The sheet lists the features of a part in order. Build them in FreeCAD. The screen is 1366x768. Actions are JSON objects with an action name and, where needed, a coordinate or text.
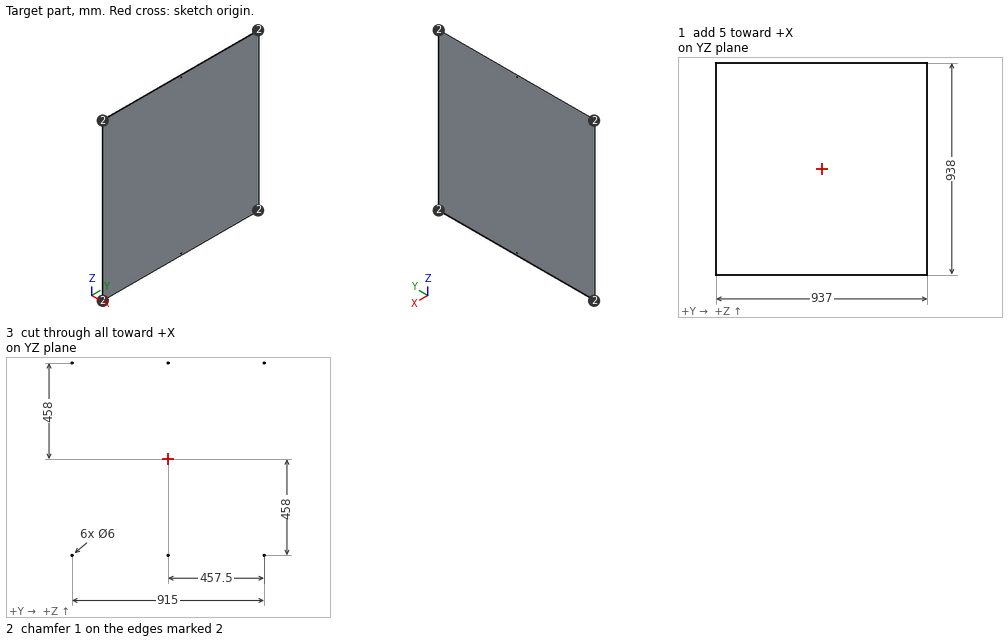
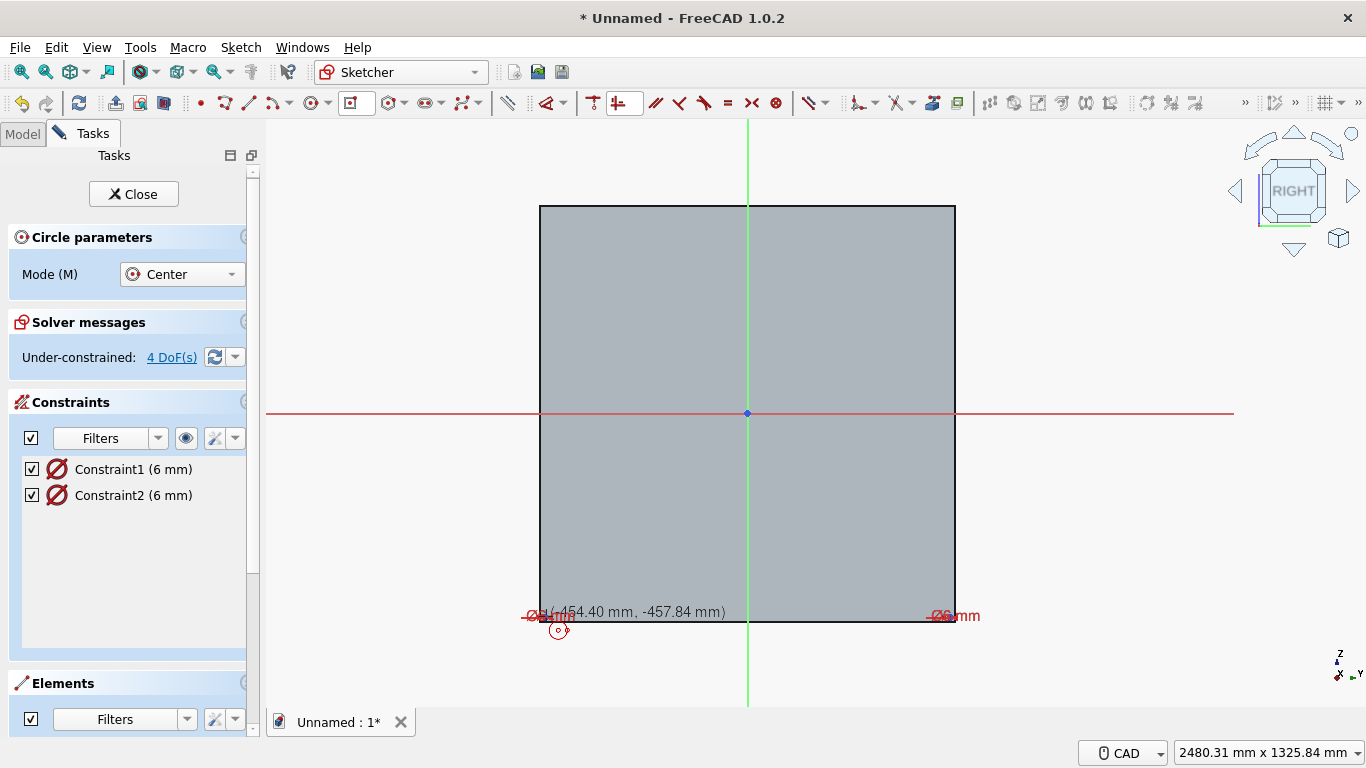
{"action": "scroll", "coordinate": [545, 211], "scroll_direction": "up", "scroll_amount": 15}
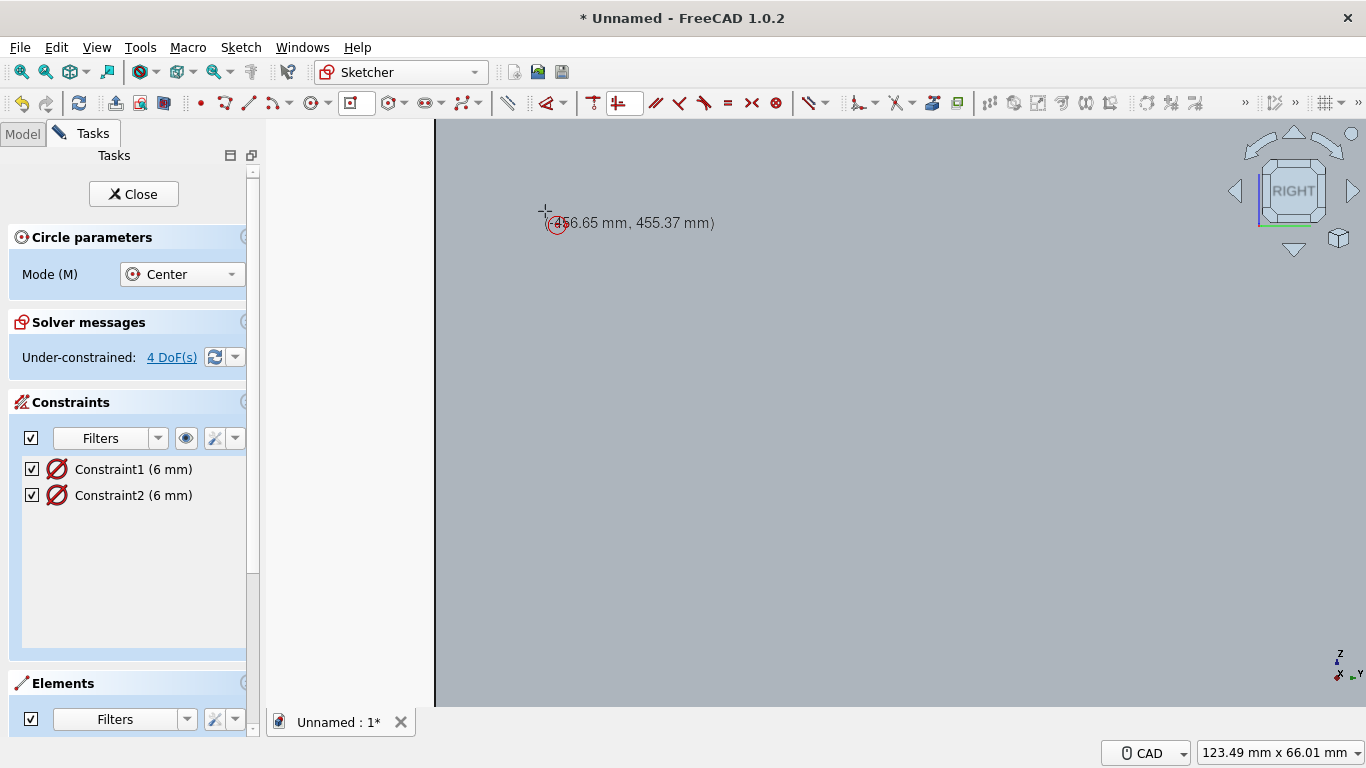
{"action": "scroll", "coordinate": [545, 210], "scroll_direction": "down", "scroll_amount": 15}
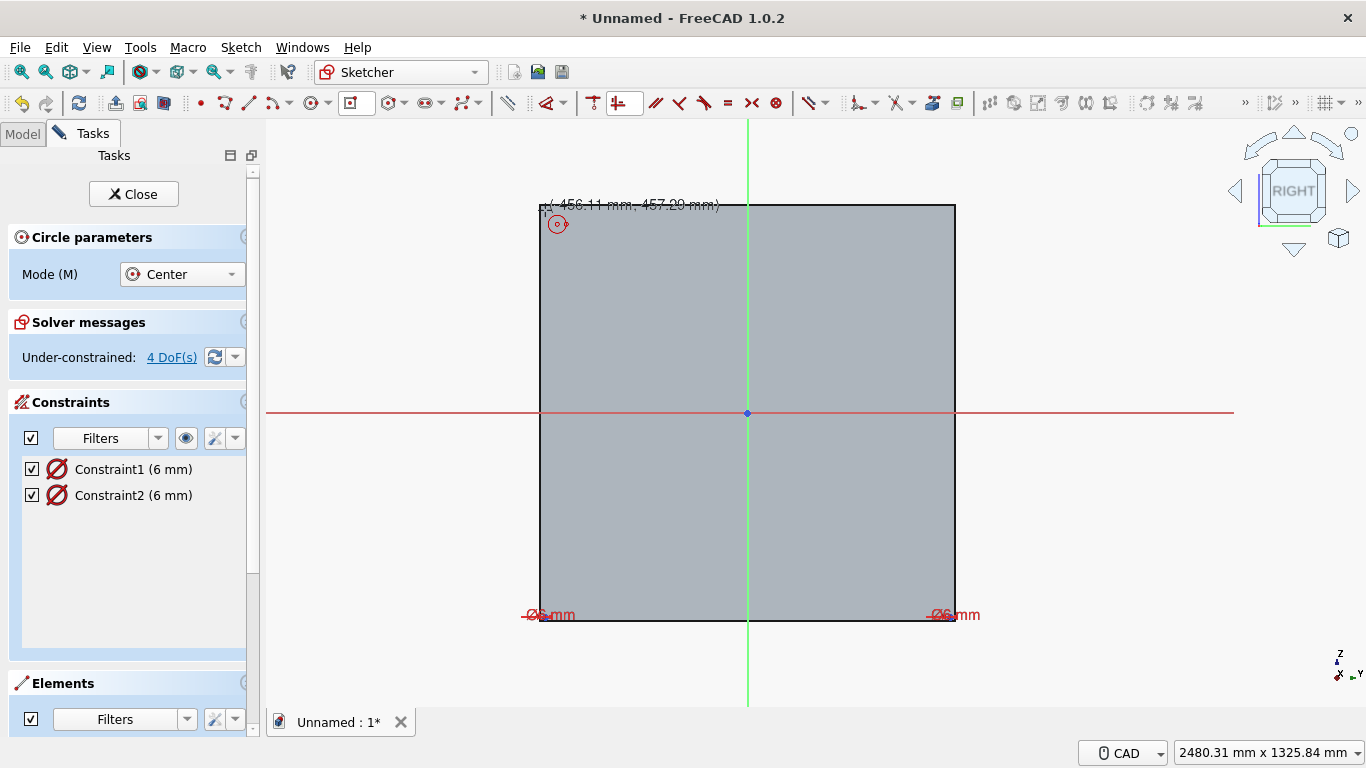
{"action": "left_click", "coordinate": [545, 210]}
{"action": "mouse_move", "coordinate": [546, 209]}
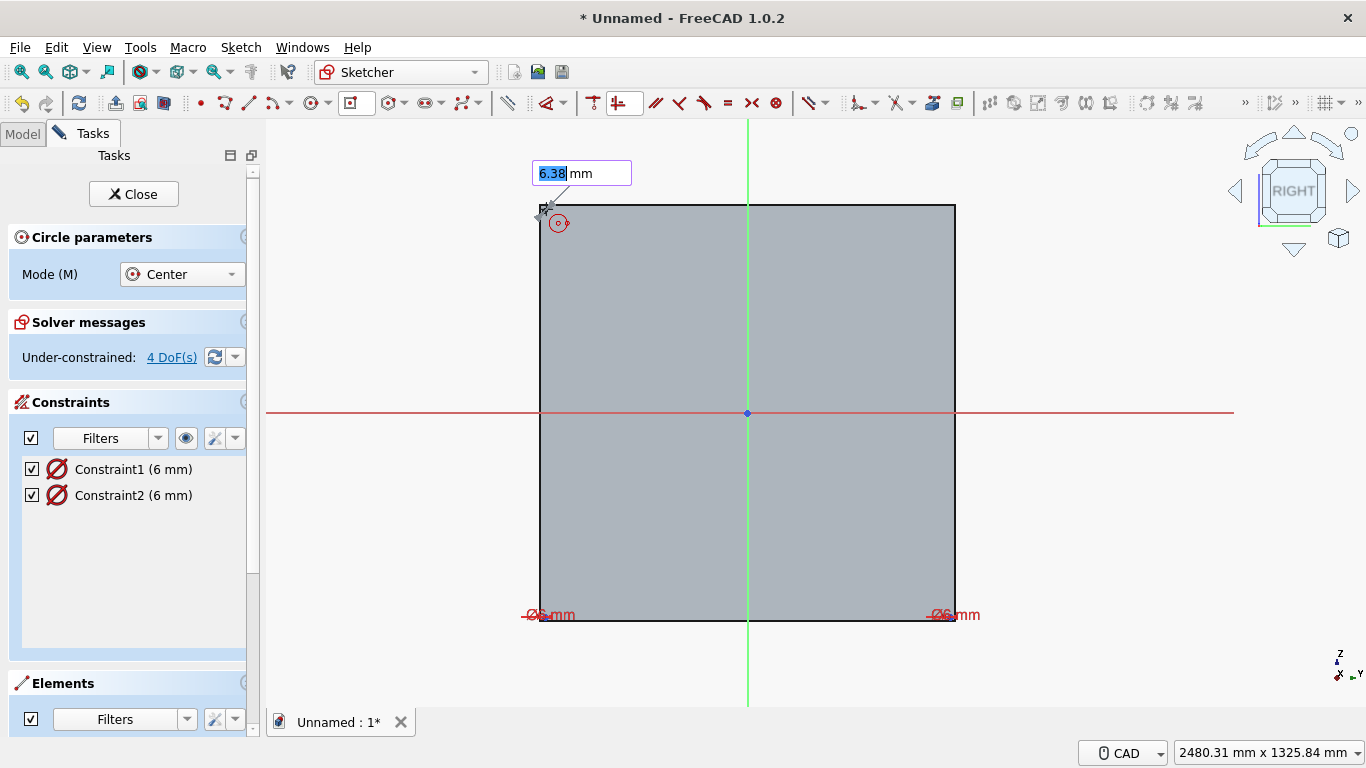
{"action": "type", "text": "6"}
{"action": "key", "text": "Return"}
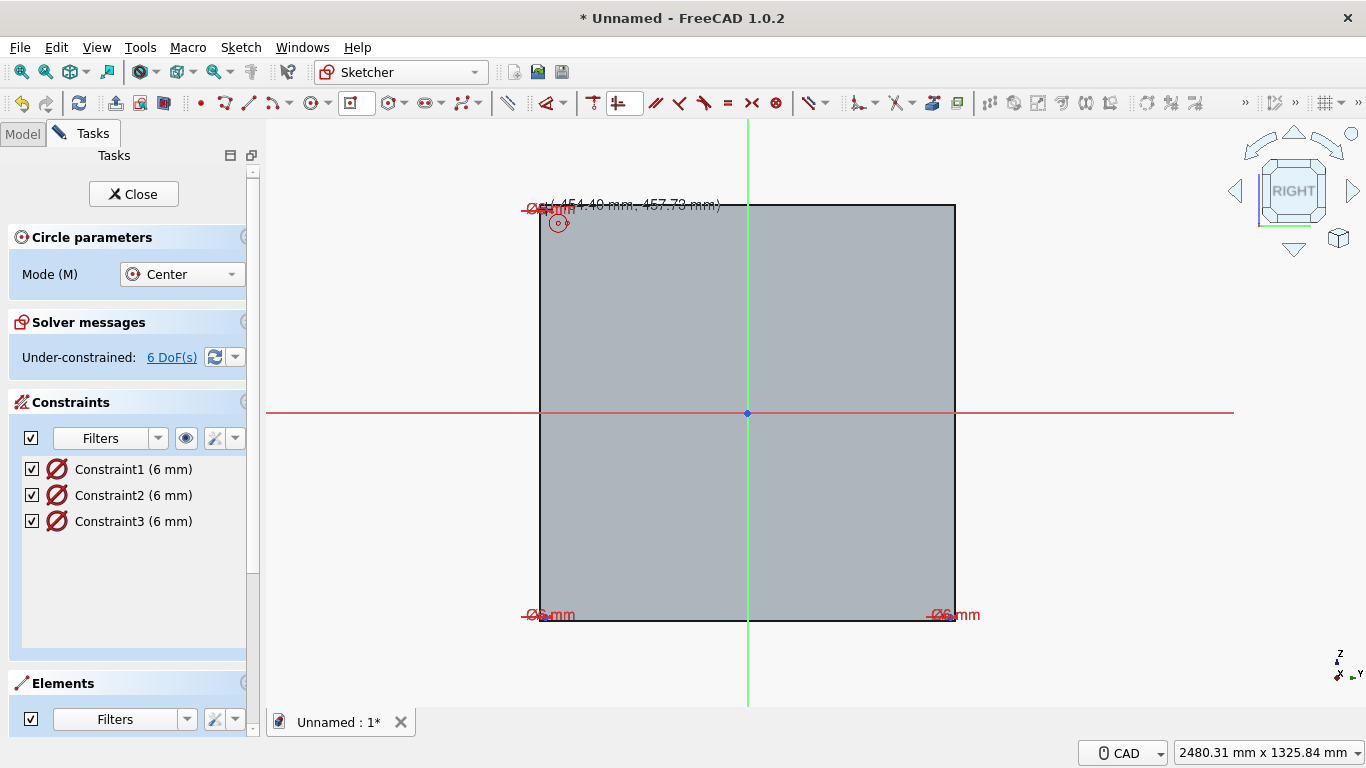
{"action": "scroll", "coordinate": [950, 210], "scroll_direction": "up", "scroll_amount": 15}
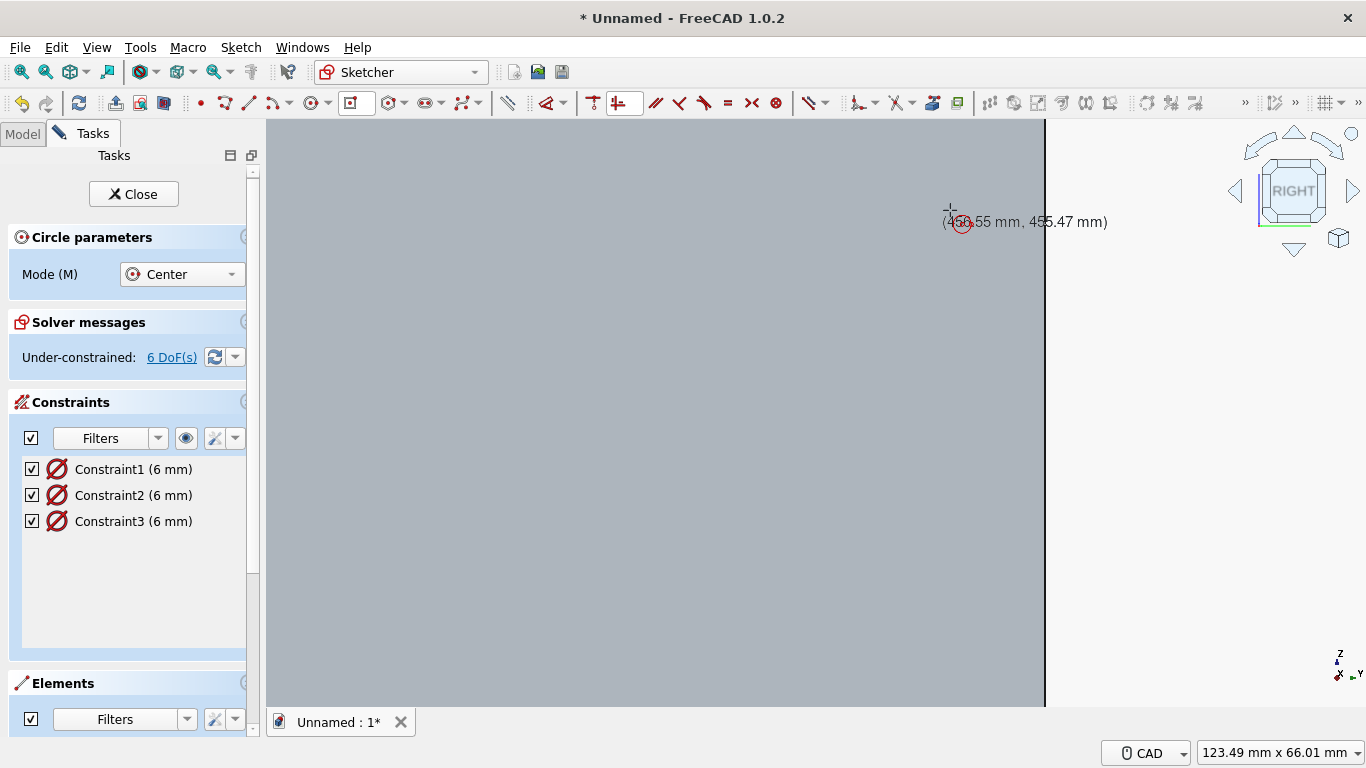
{"action": "scroll", "coordinate": [951, 210], "scroll_direction": "down", "scroll_amount": 15}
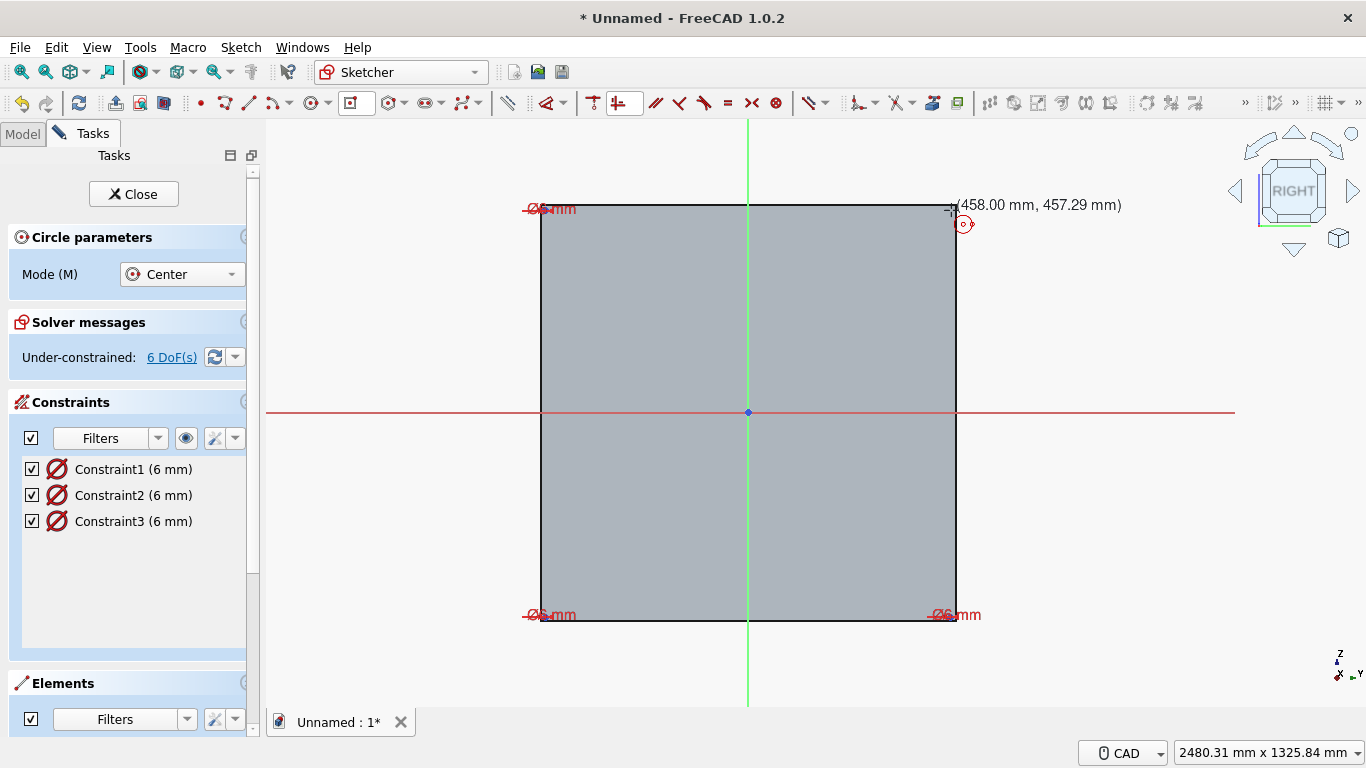
{"action": "left_click", "coordinate": [951, 210]}
{"action": "mouse_move", "coordinate": [952, 209]}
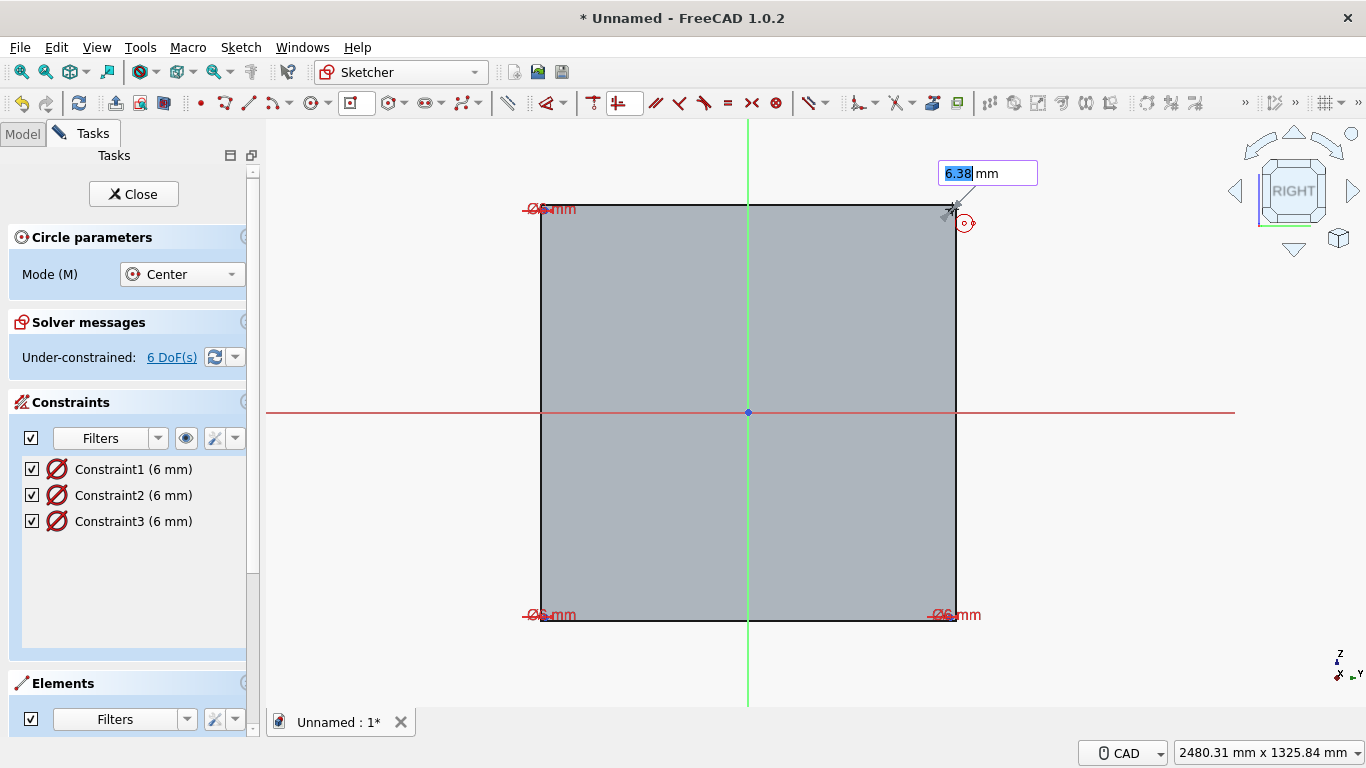
{"action": "type", "text": "6"}
{"action": "key", "text": "Return"}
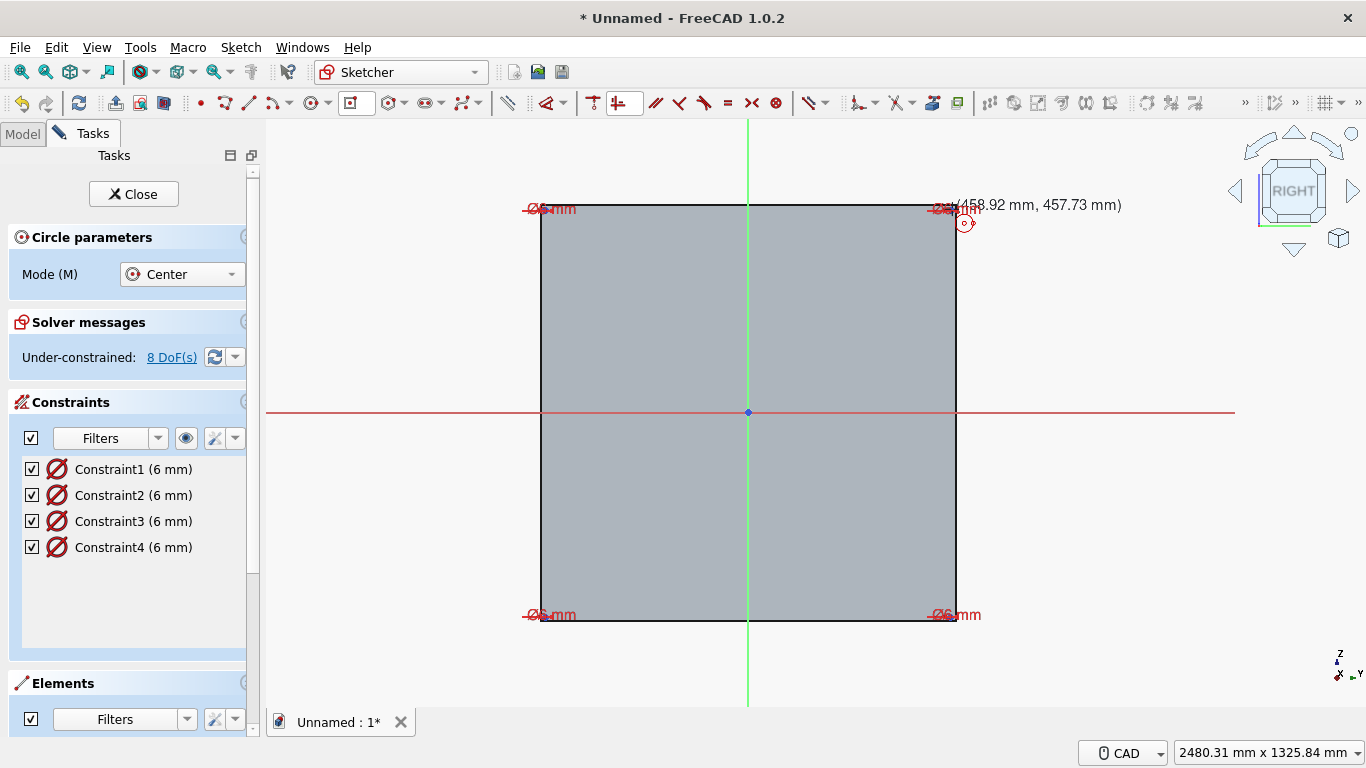
{"action": "scroll", "coordinate": [748, 210], "scroll_direction": "up", "scroll_amount": 15}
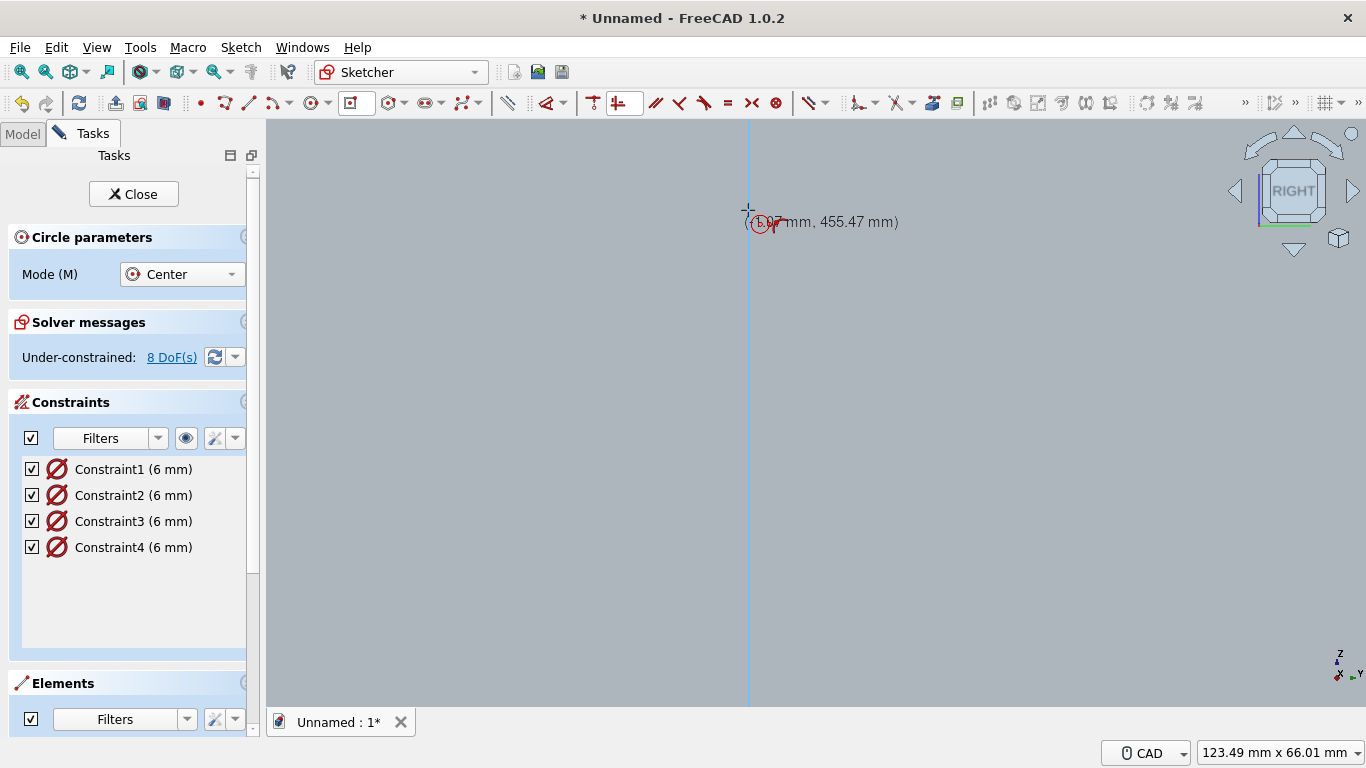
{"action": "scroll", "coordinate": [747, 210], "scroll_direction": "down", "scroll_amount": 15}